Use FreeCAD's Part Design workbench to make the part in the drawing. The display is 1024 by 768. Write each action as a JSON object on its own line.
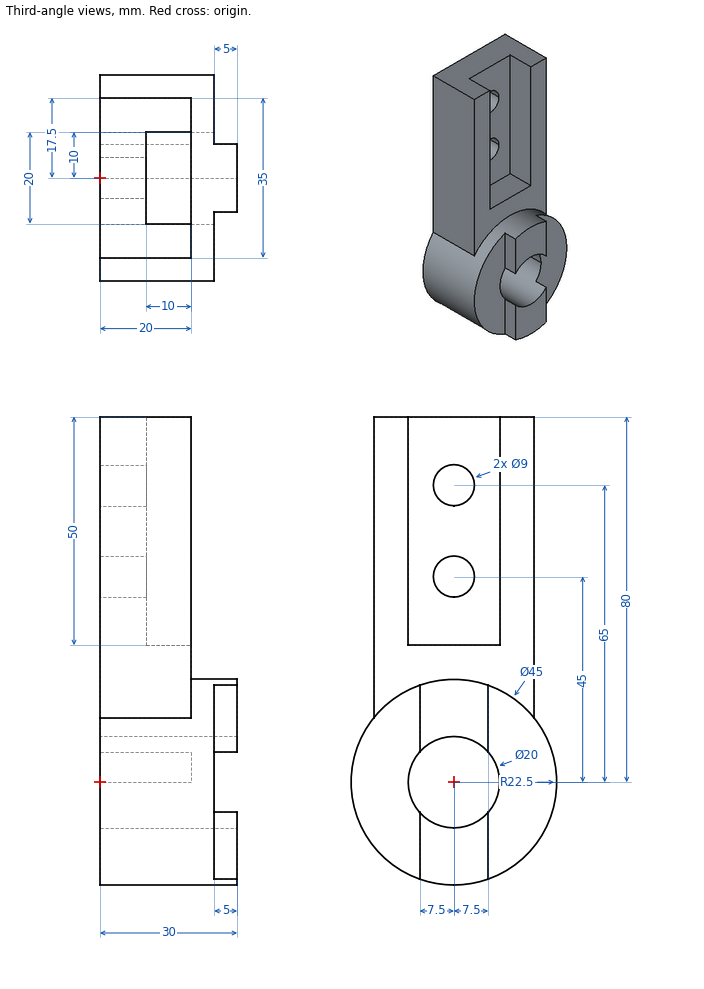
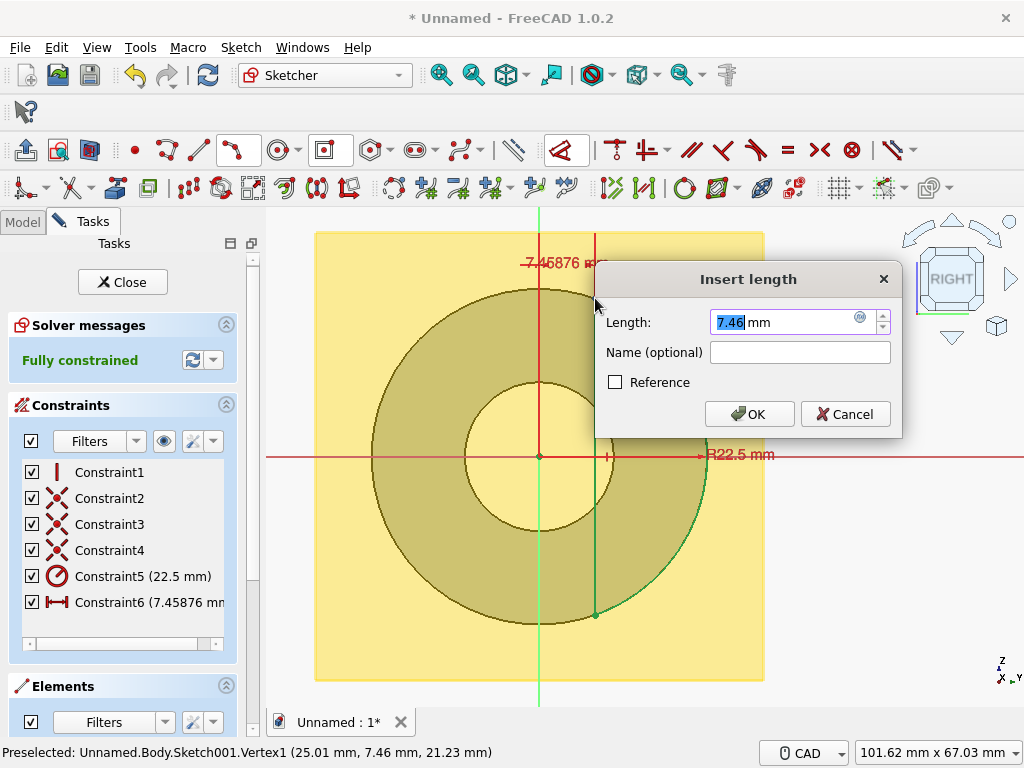
{"action": "type", "text": "7.5"}
{"action": "key", "text": "Return"}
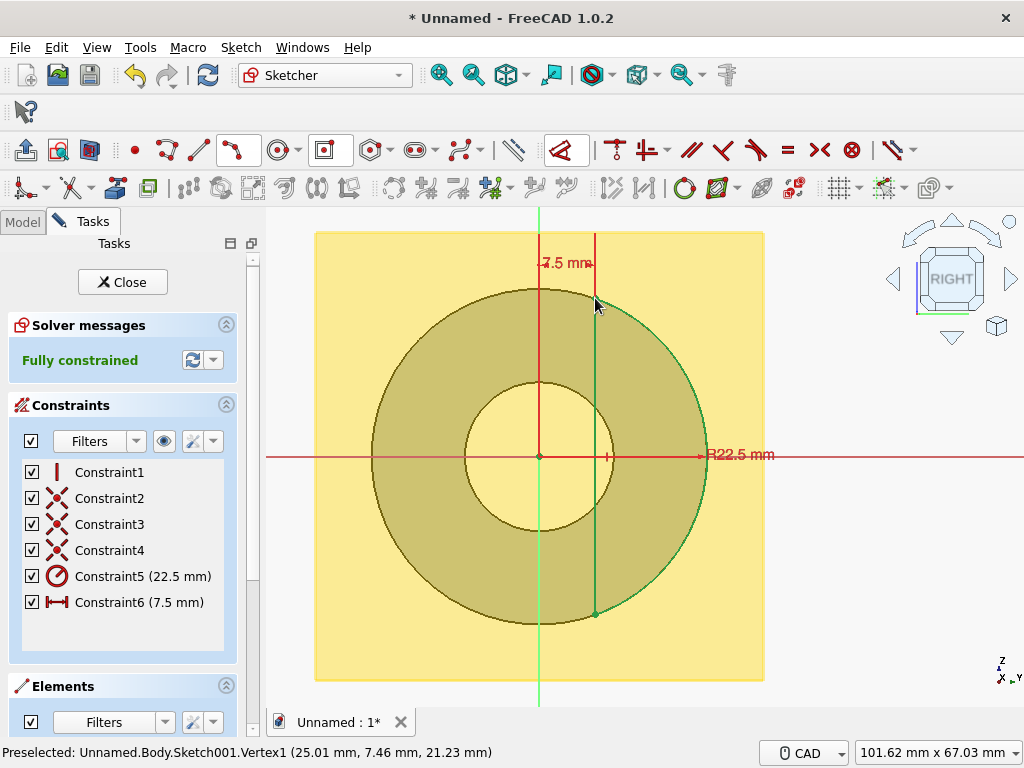
{"action": "left_click", "coordinate": [123, 282]}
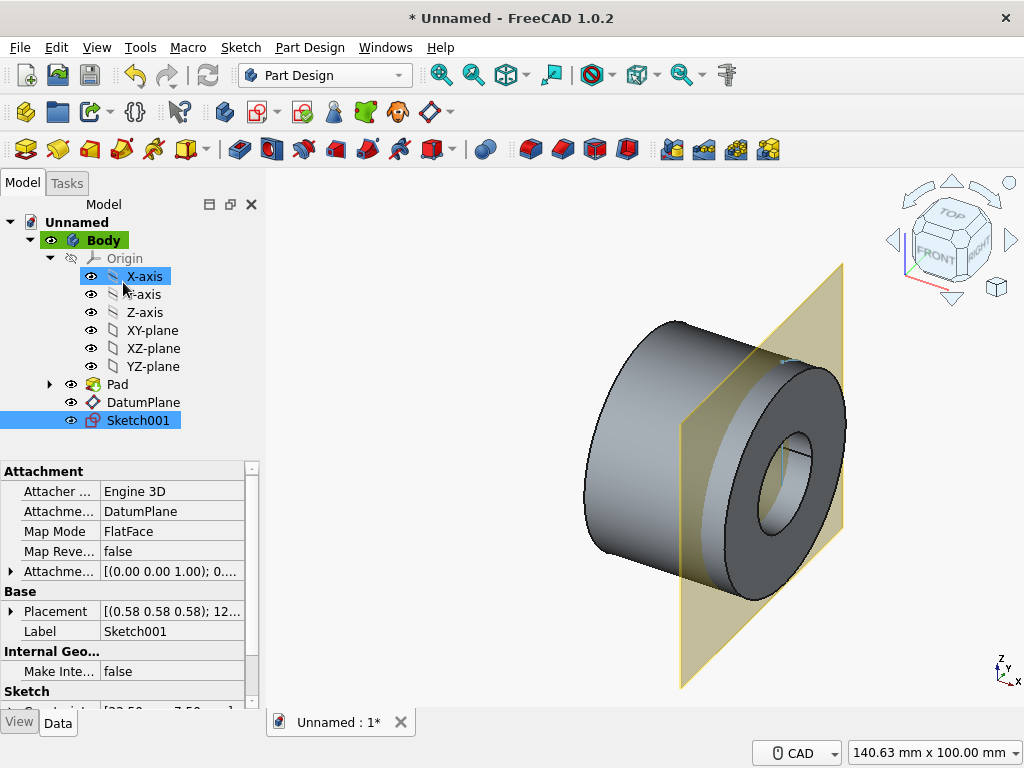
{"action": "left_click", "coordinate": [240, 150]}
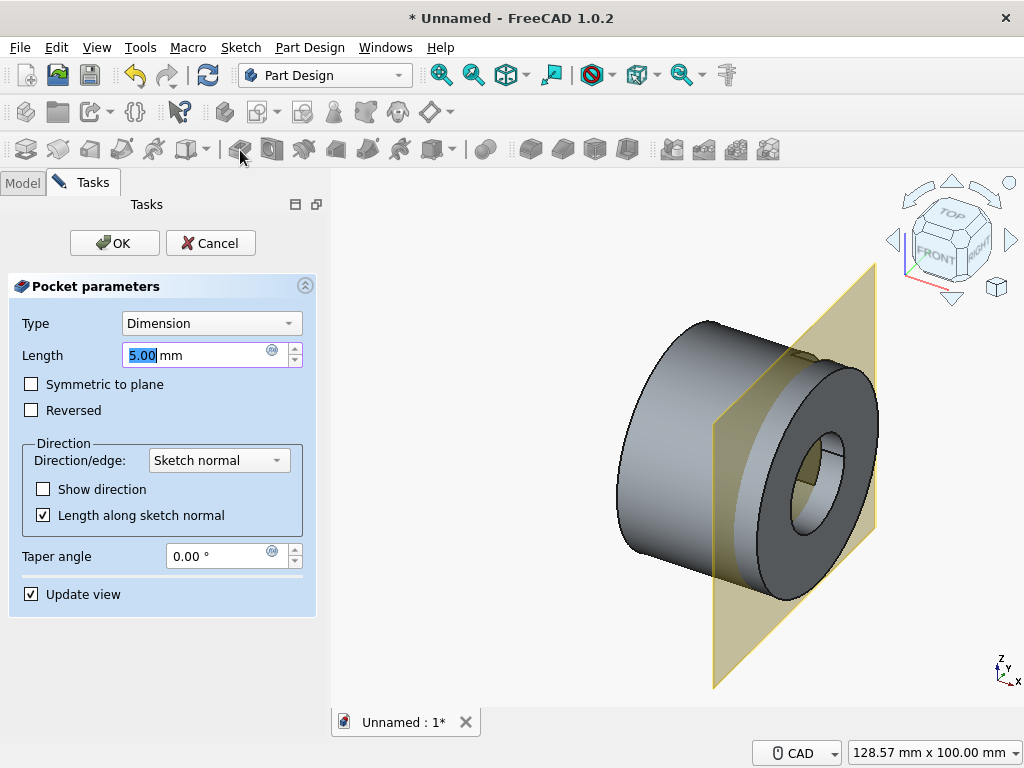
{"action": "type", "text": "5"}
{"action": "key", "text": "Tab"}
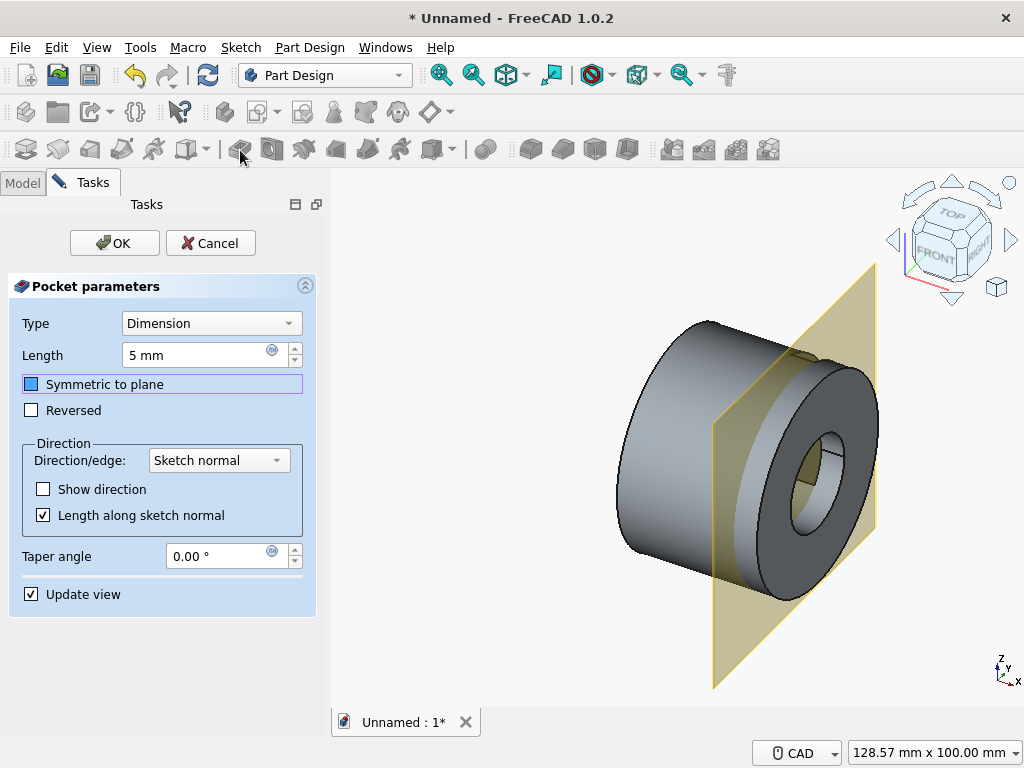
{"action": "left_click", "coordinate": [30, 410]}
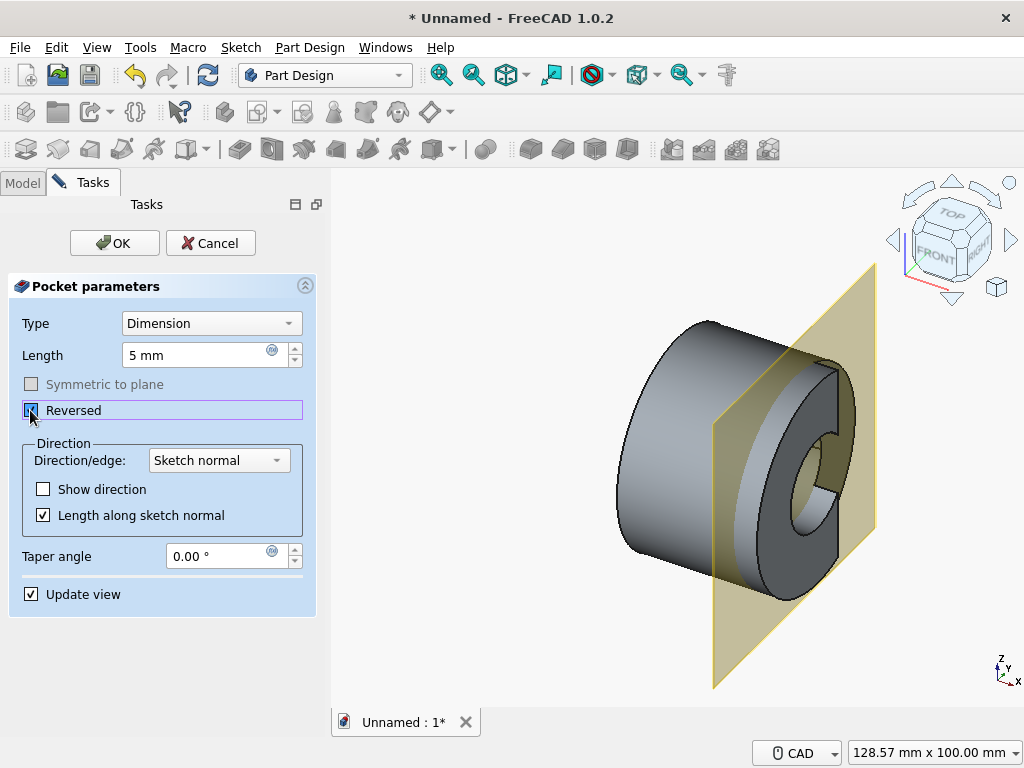
{"action": "left_click", "coordinate": [115, 243]}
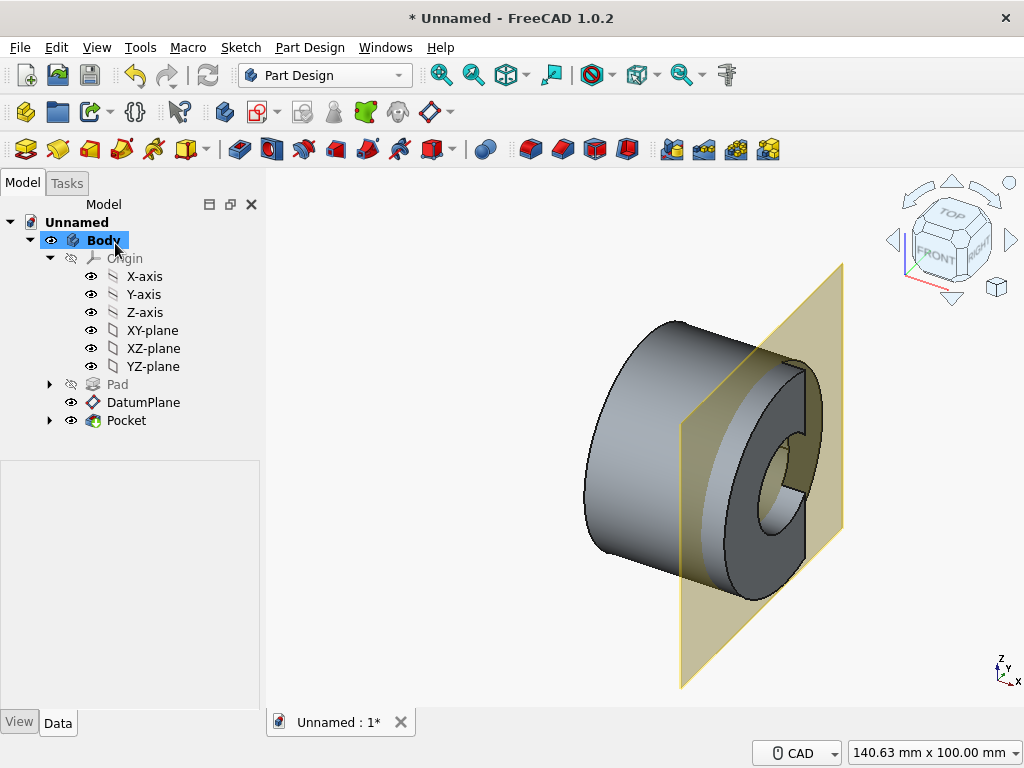
{"action": "left_click", "coordinate": [116, 402]}
{"action": "key", "text": "space"}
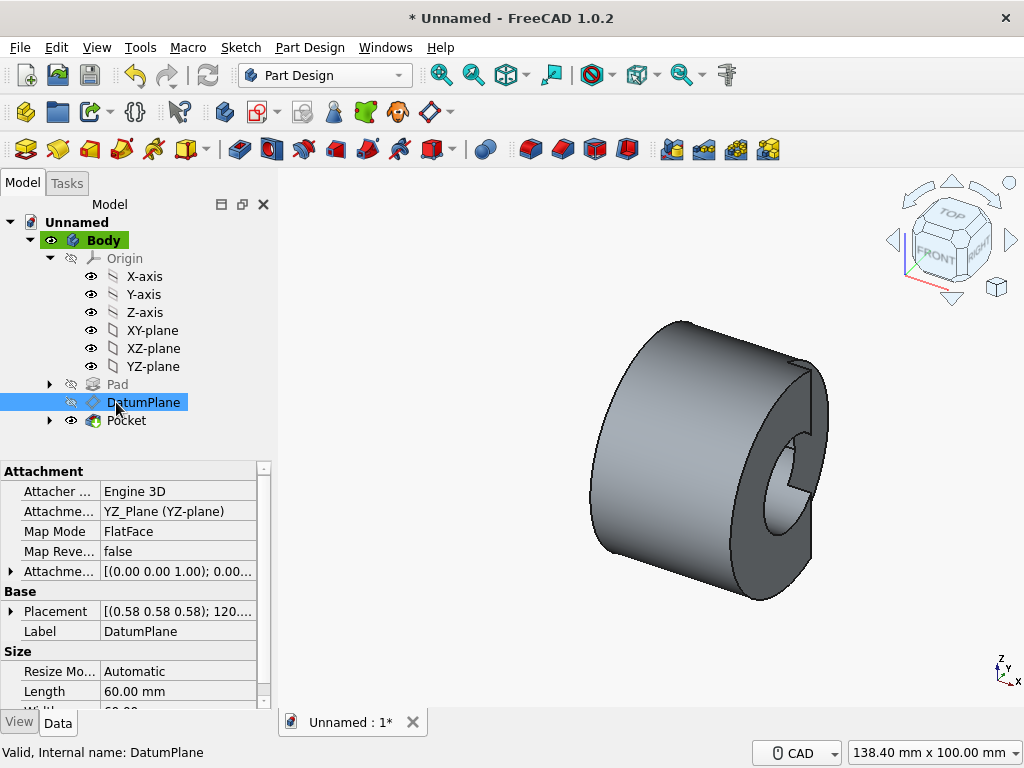
{"action": "left_click", "coordinate": [808, 462]}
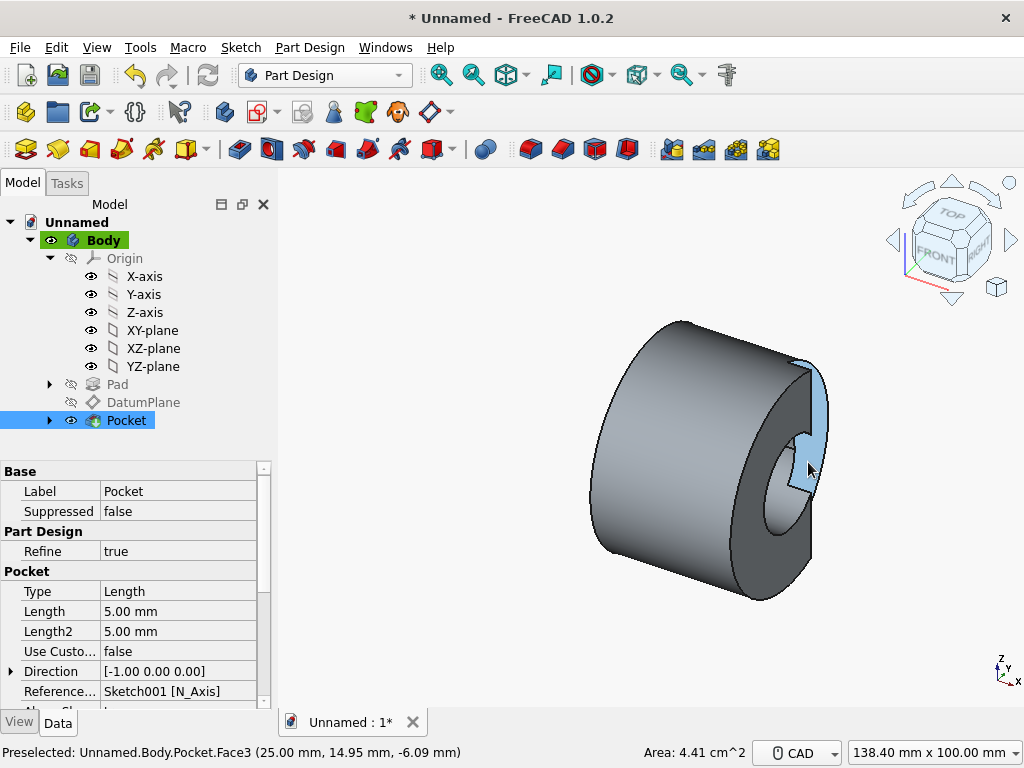
{"action": "left_click", "coordinate": [258, 112]}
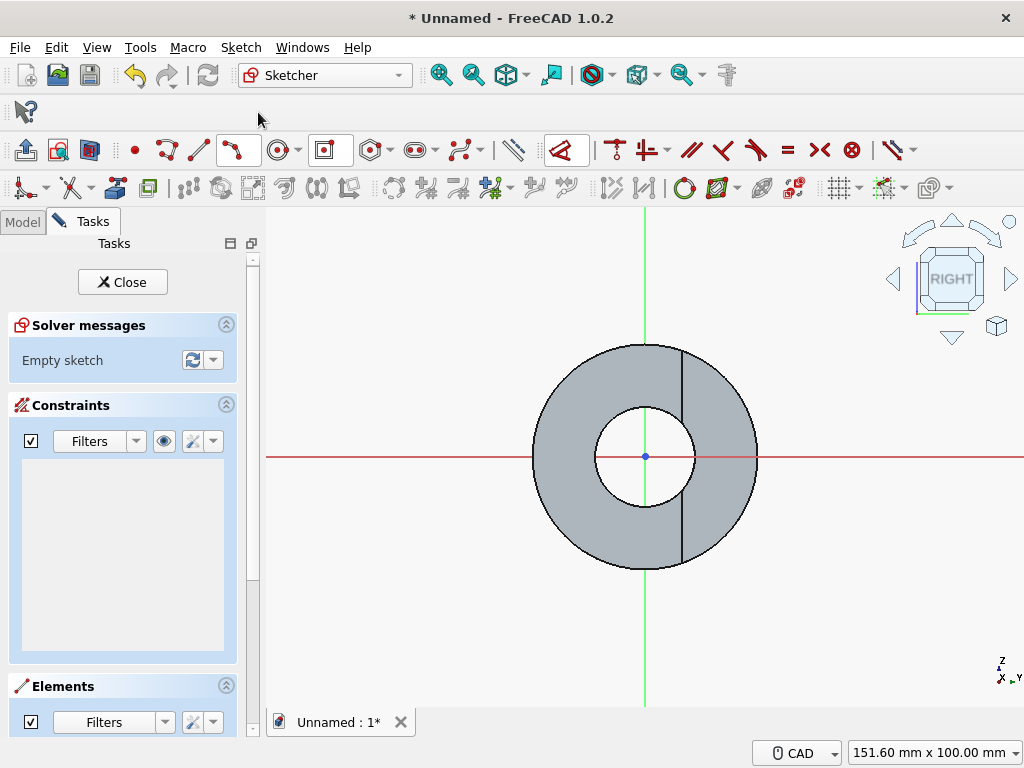
{"action": "scroll", "coordinate": [614, 457], "scroll_direction": "up", "scroll_amount": 2}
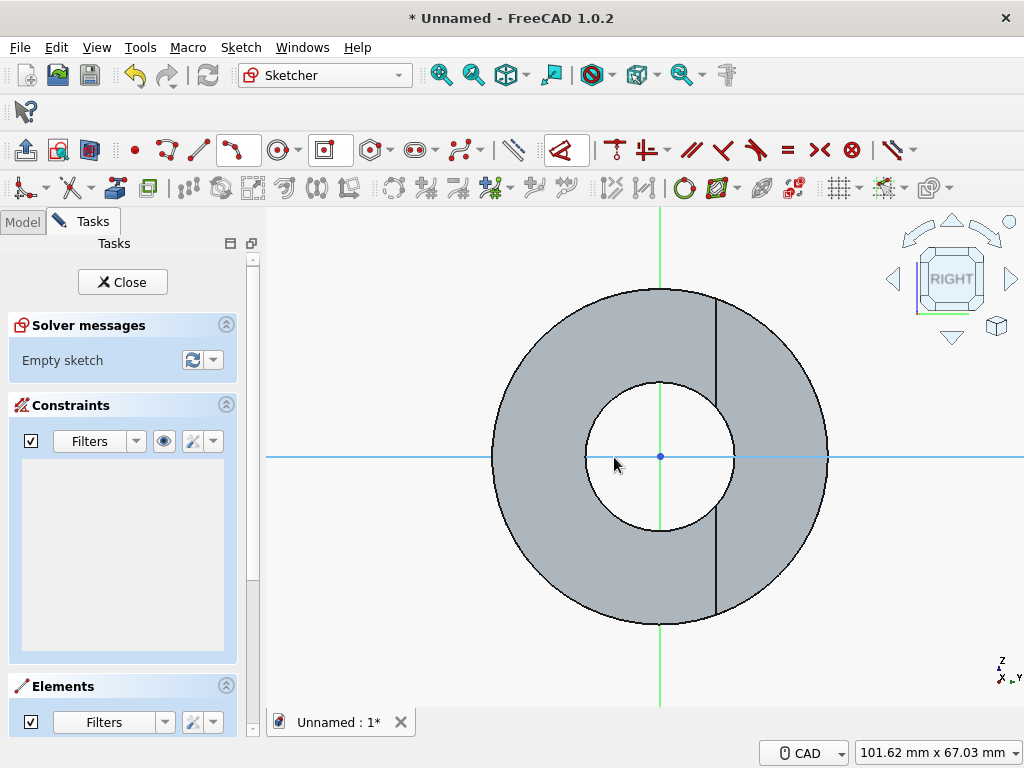
{"action": "left_click", "coordinate": [200, 150]}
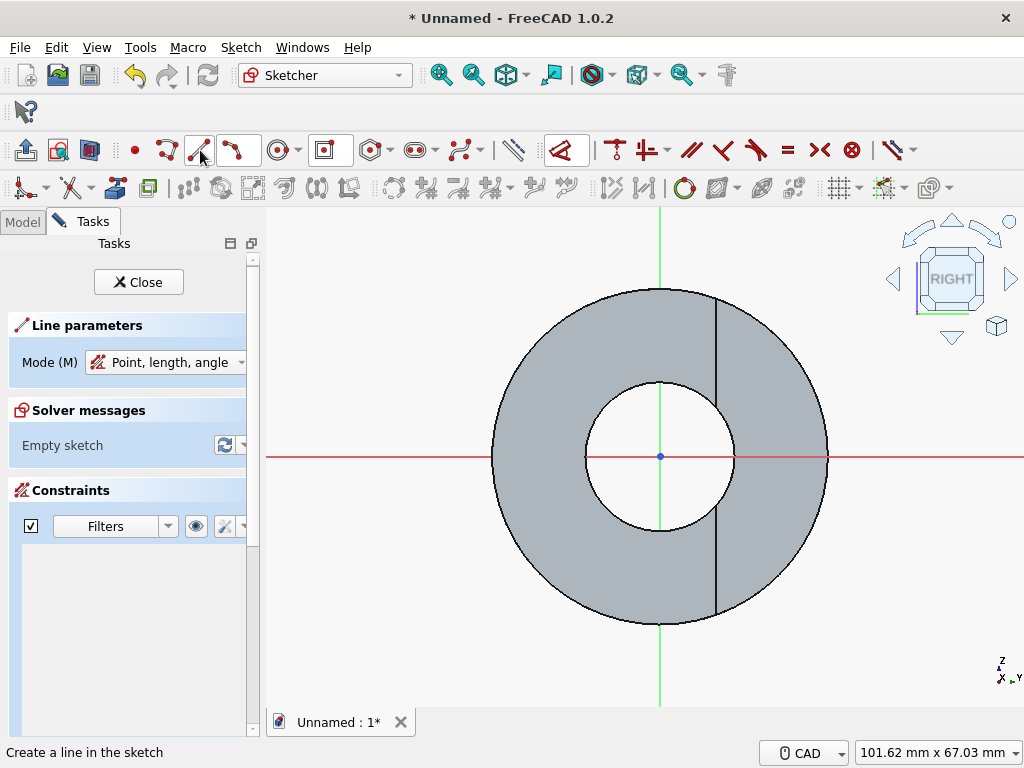
{"action": "left_click", "coordinate": [604, 615]}
{"action": "left_click", "coordinate": [604, 299]}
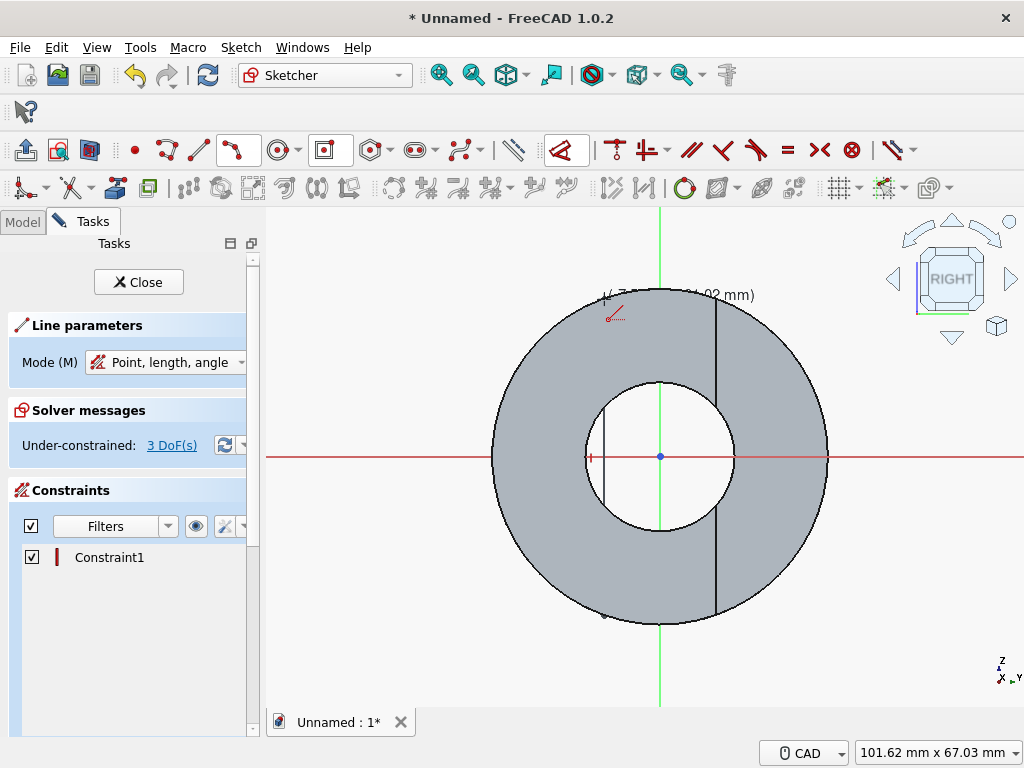
{"action": "left_click", "coordinate": [232, 150]}